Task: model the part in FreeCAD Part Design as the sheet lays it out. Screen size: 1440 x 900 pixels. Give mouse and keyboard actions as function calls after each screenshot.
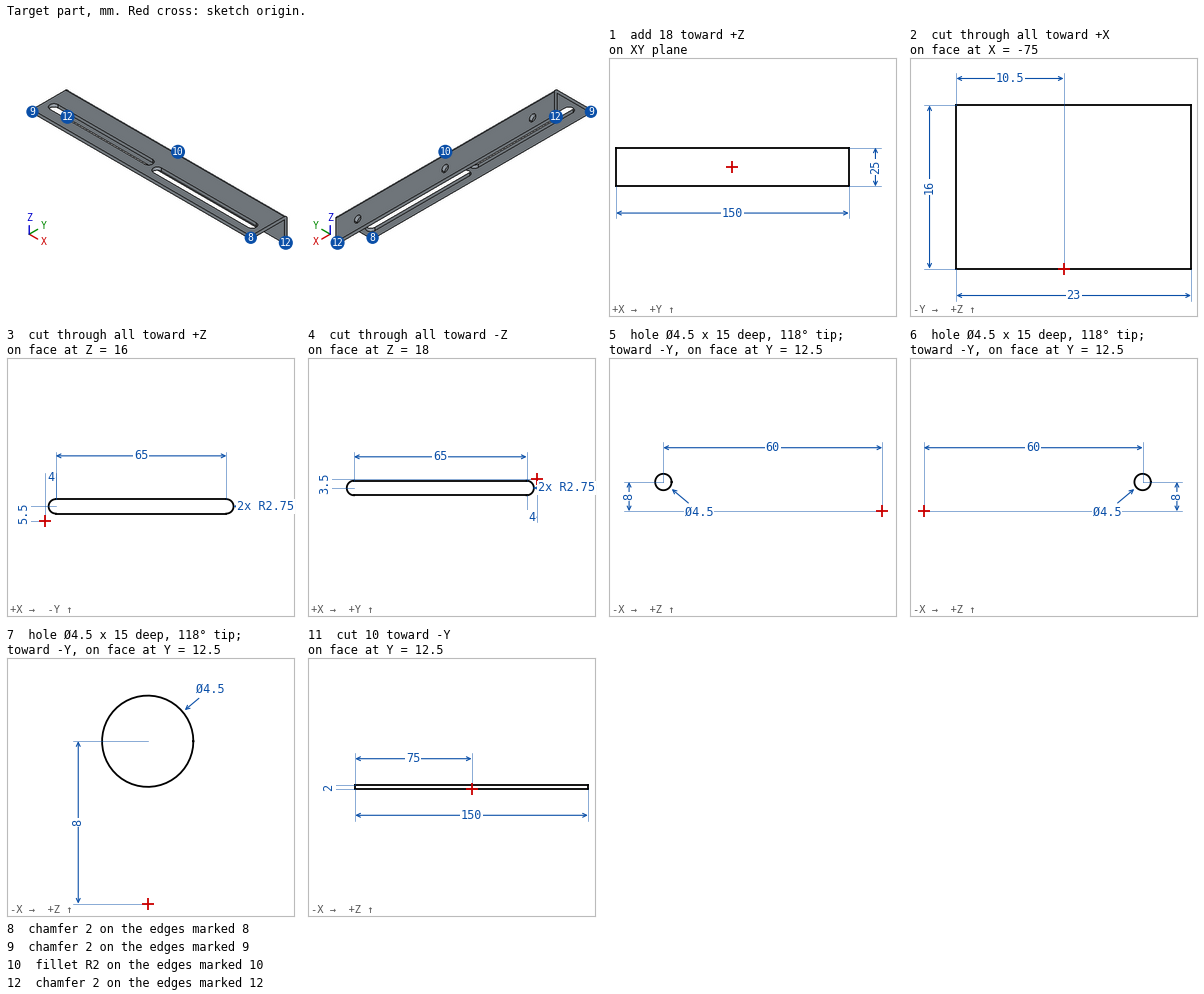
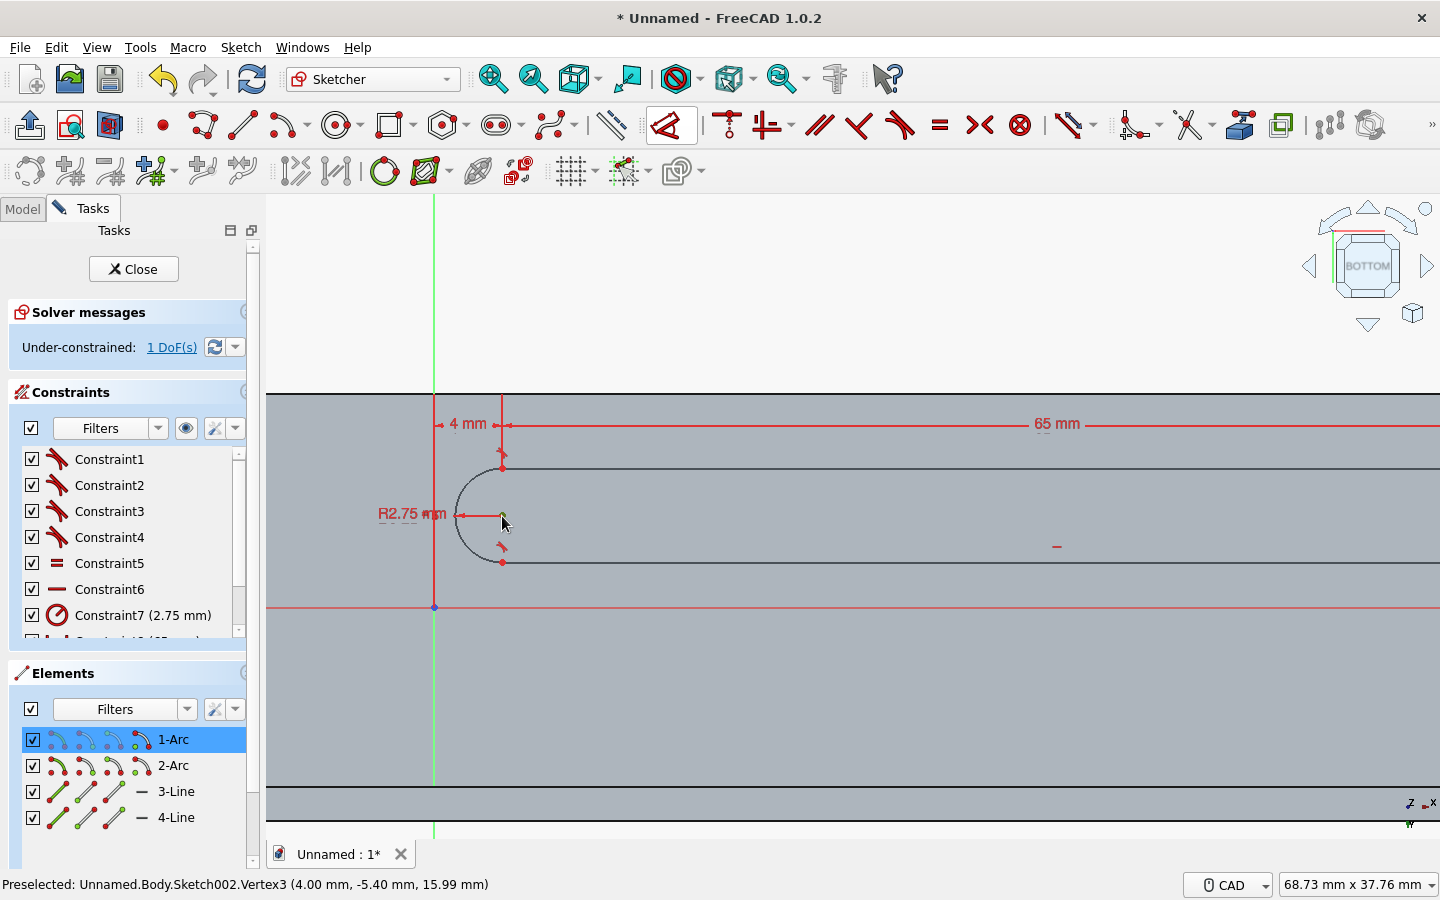
click(692, 126)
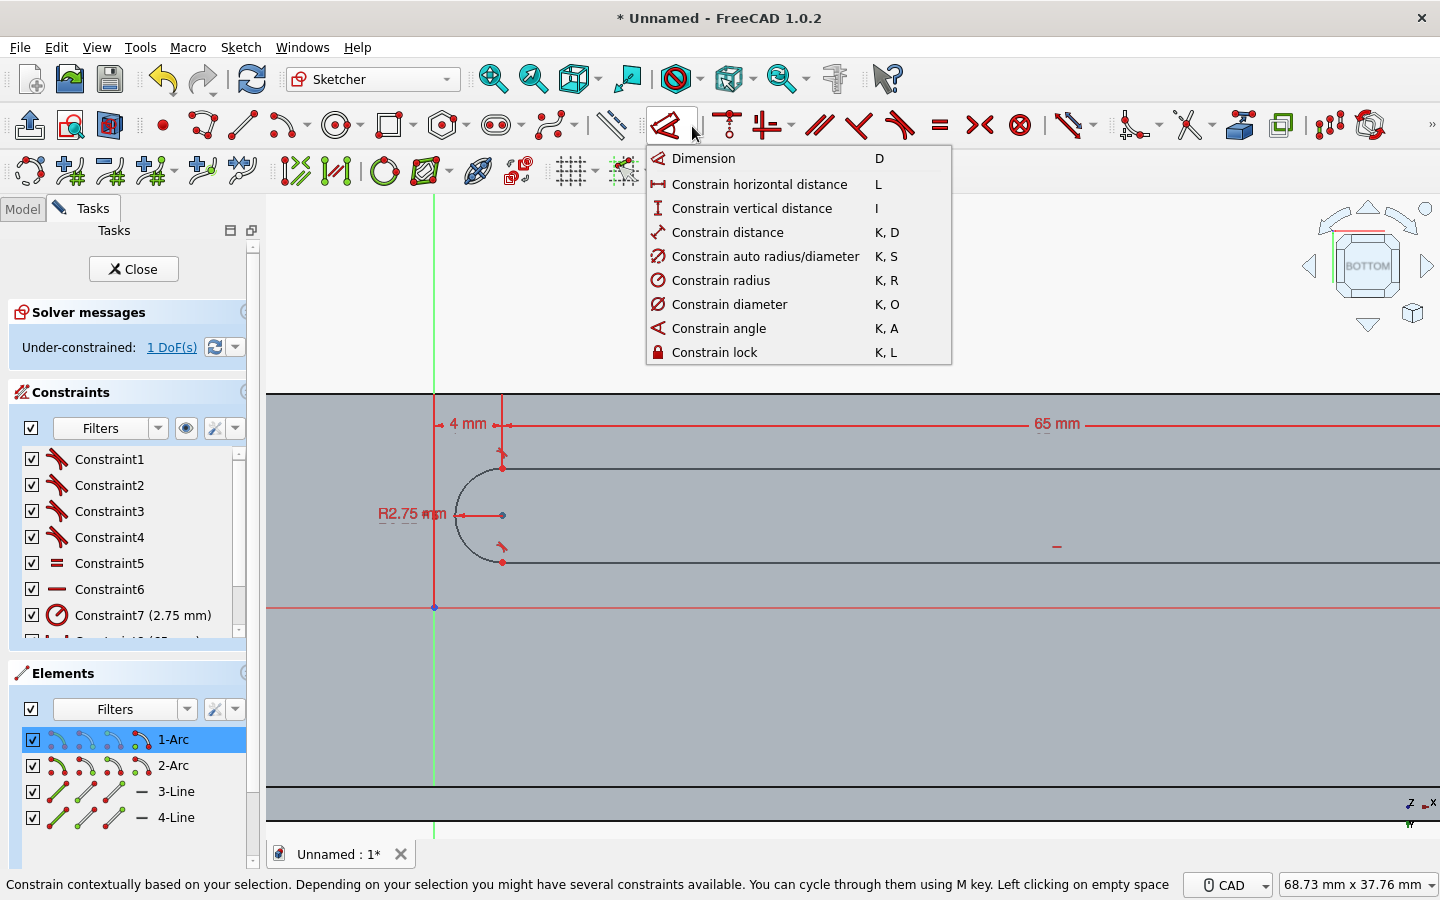
click(799, 208)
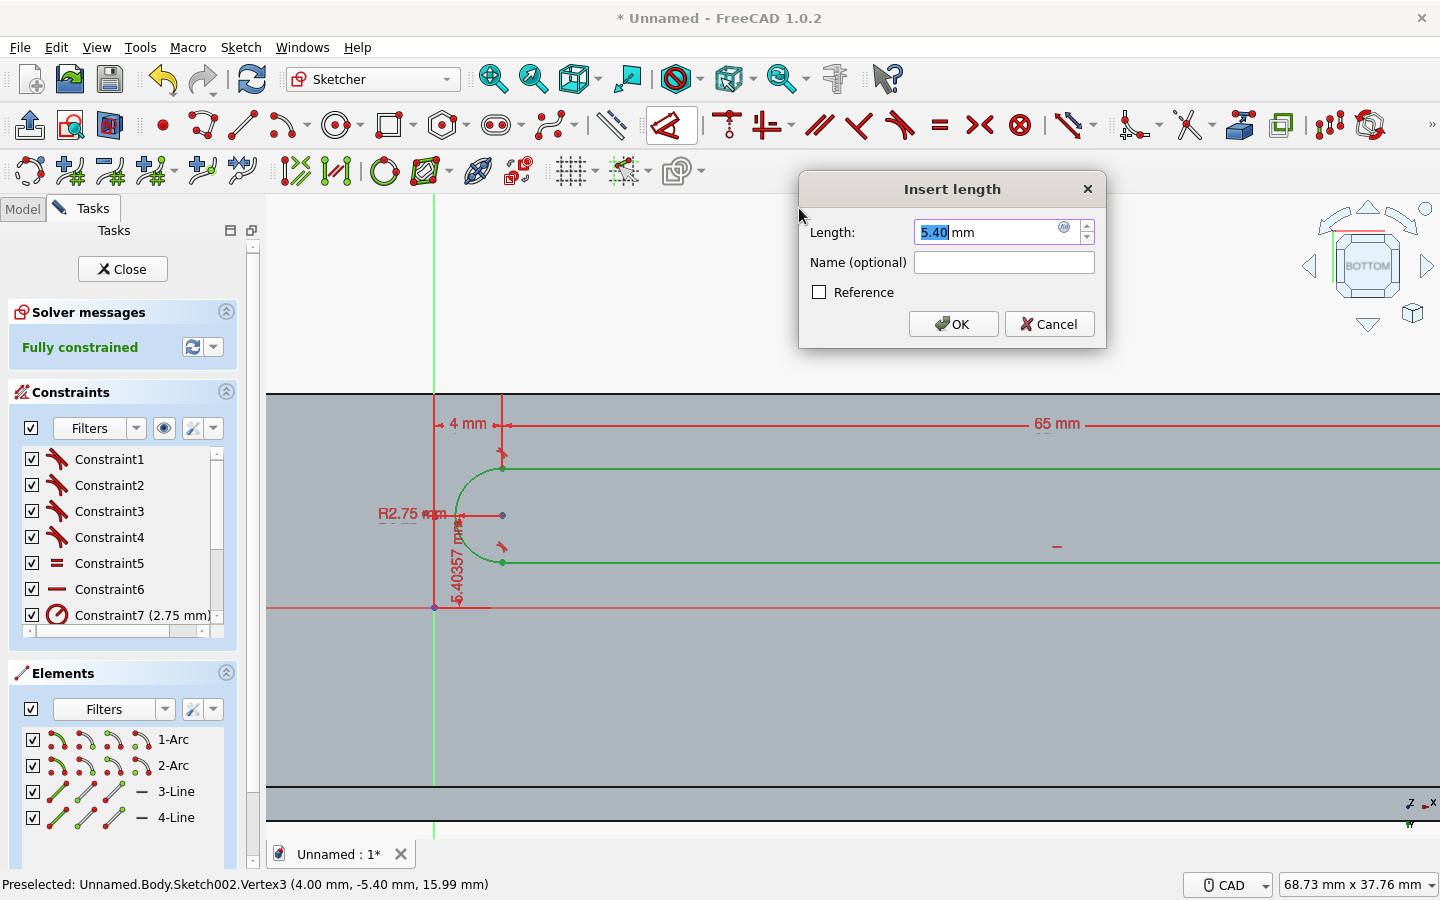
text(5.5)
key(Return)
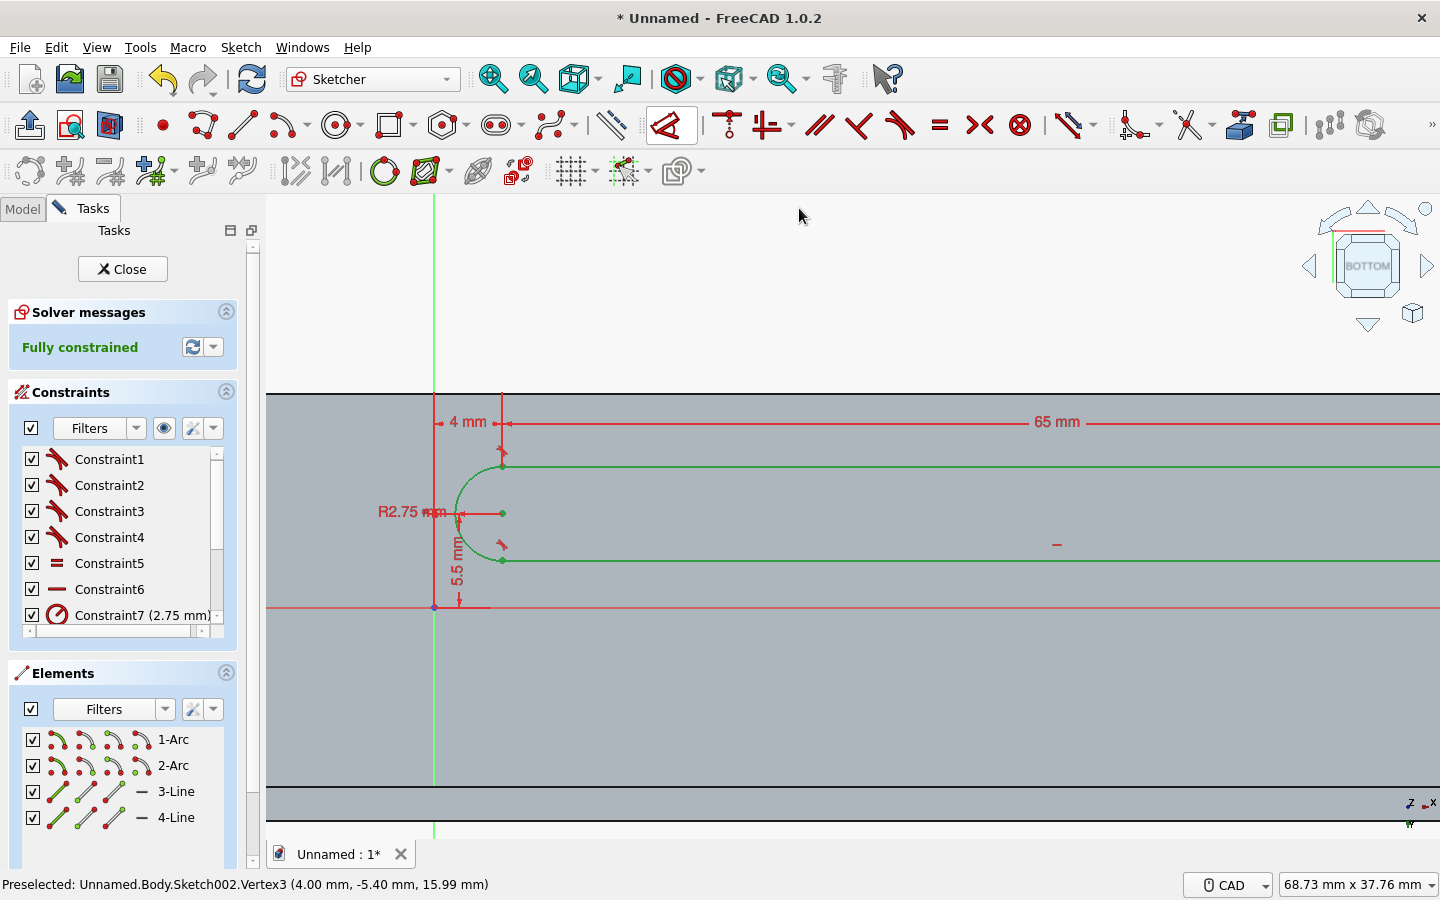
click(123, 269)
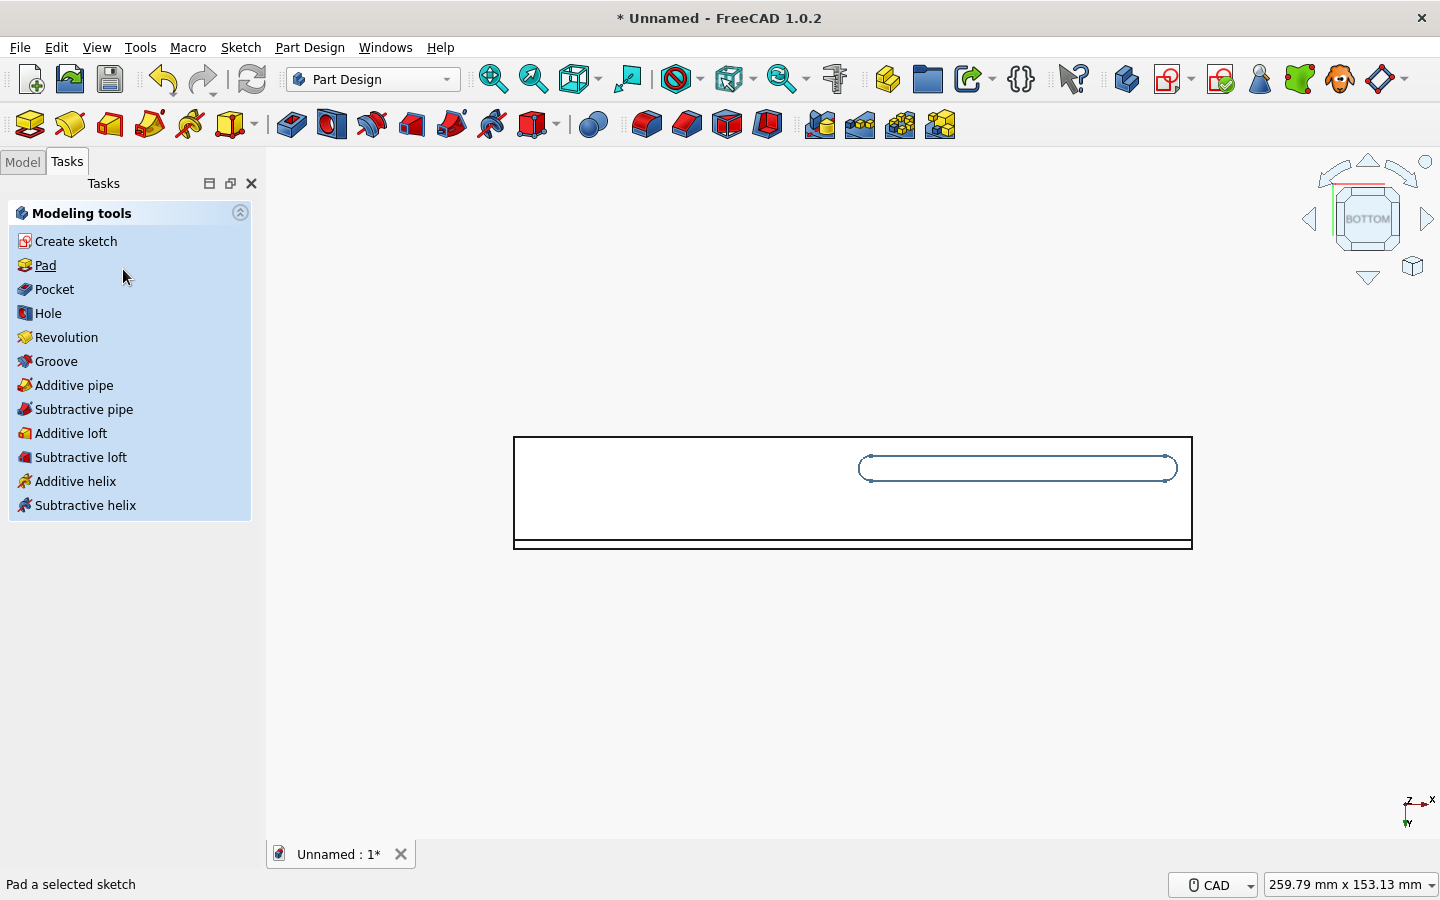
click(292, 124)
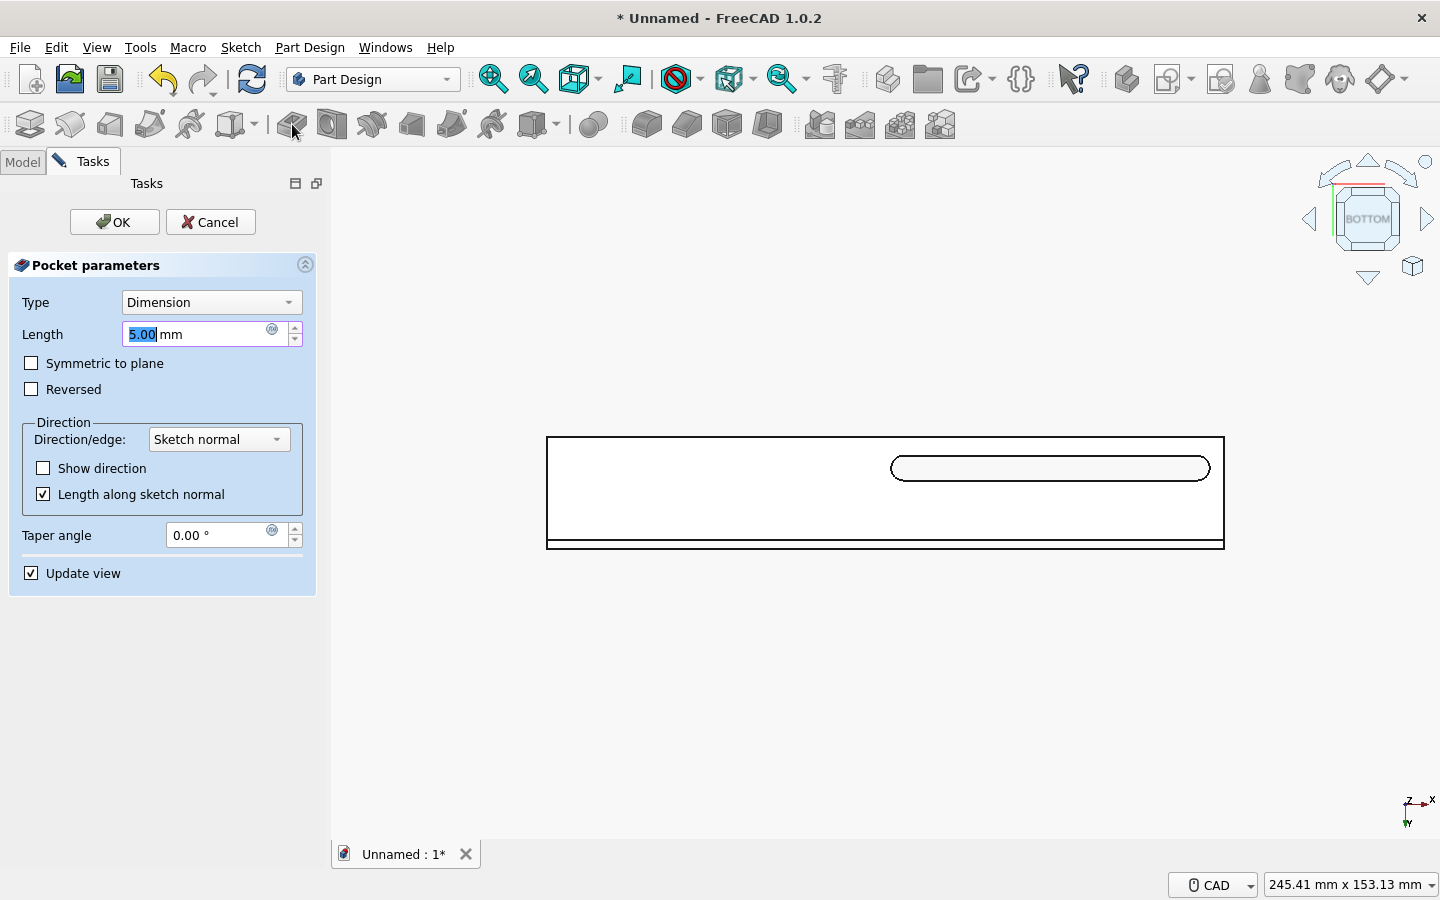
click(212, 302)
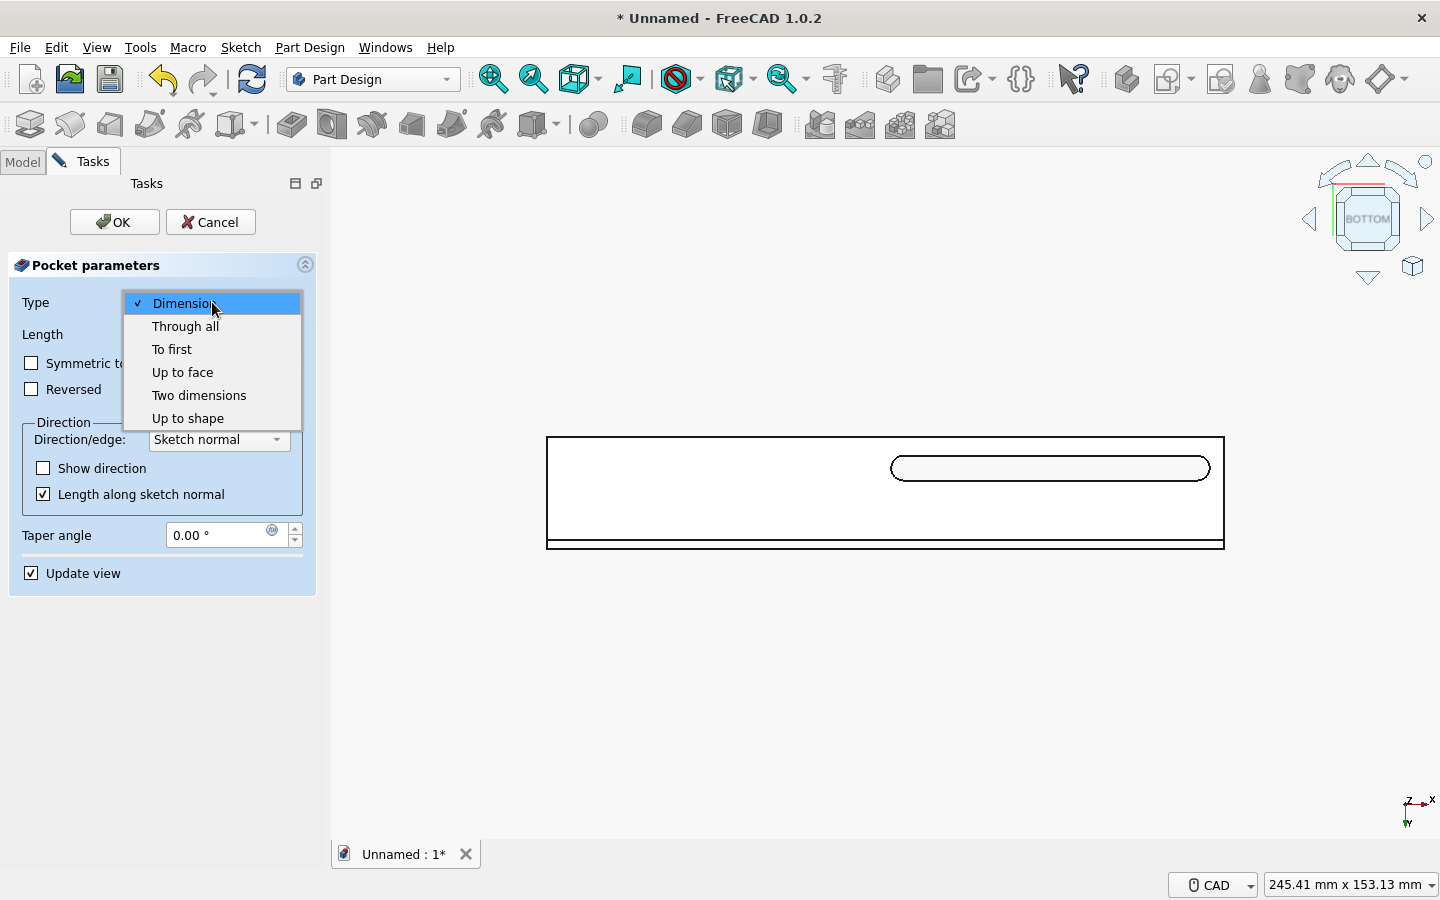
click(212, 326)